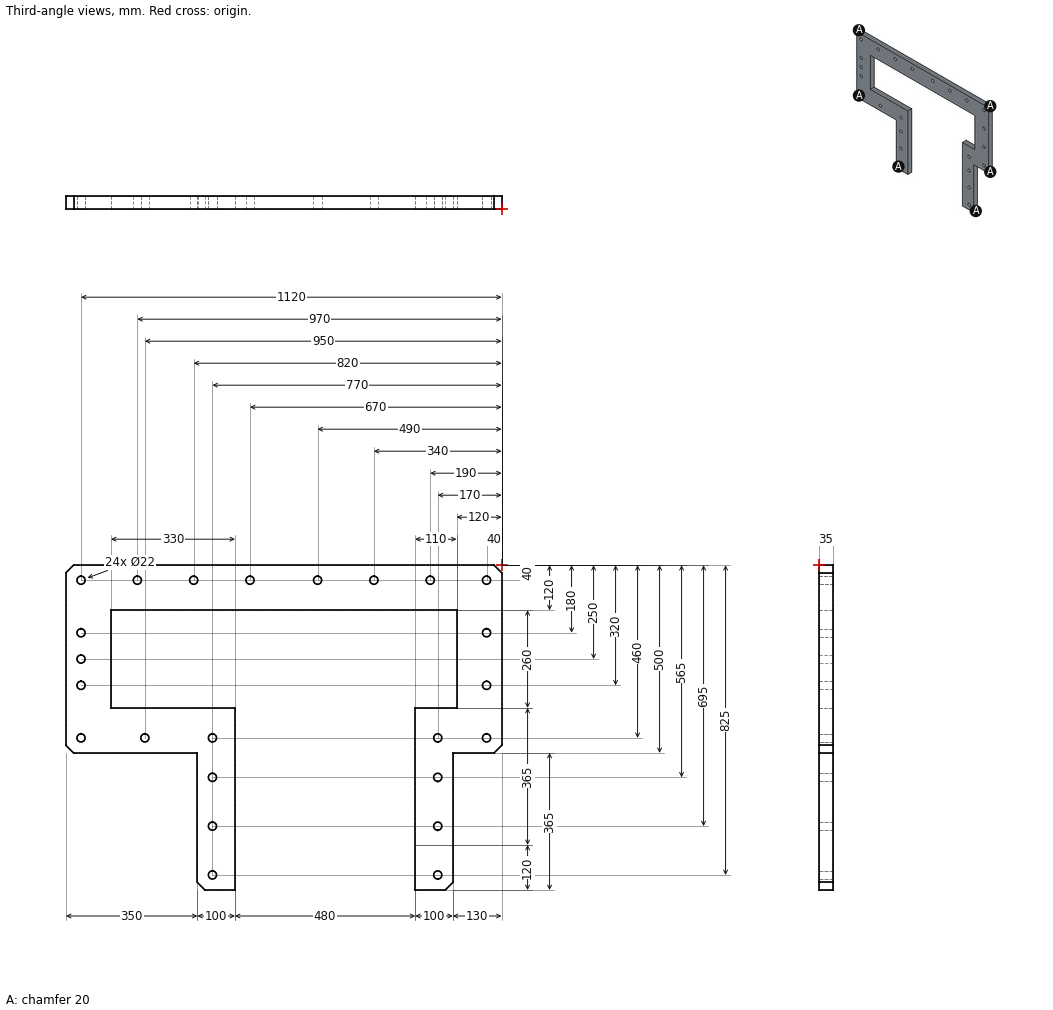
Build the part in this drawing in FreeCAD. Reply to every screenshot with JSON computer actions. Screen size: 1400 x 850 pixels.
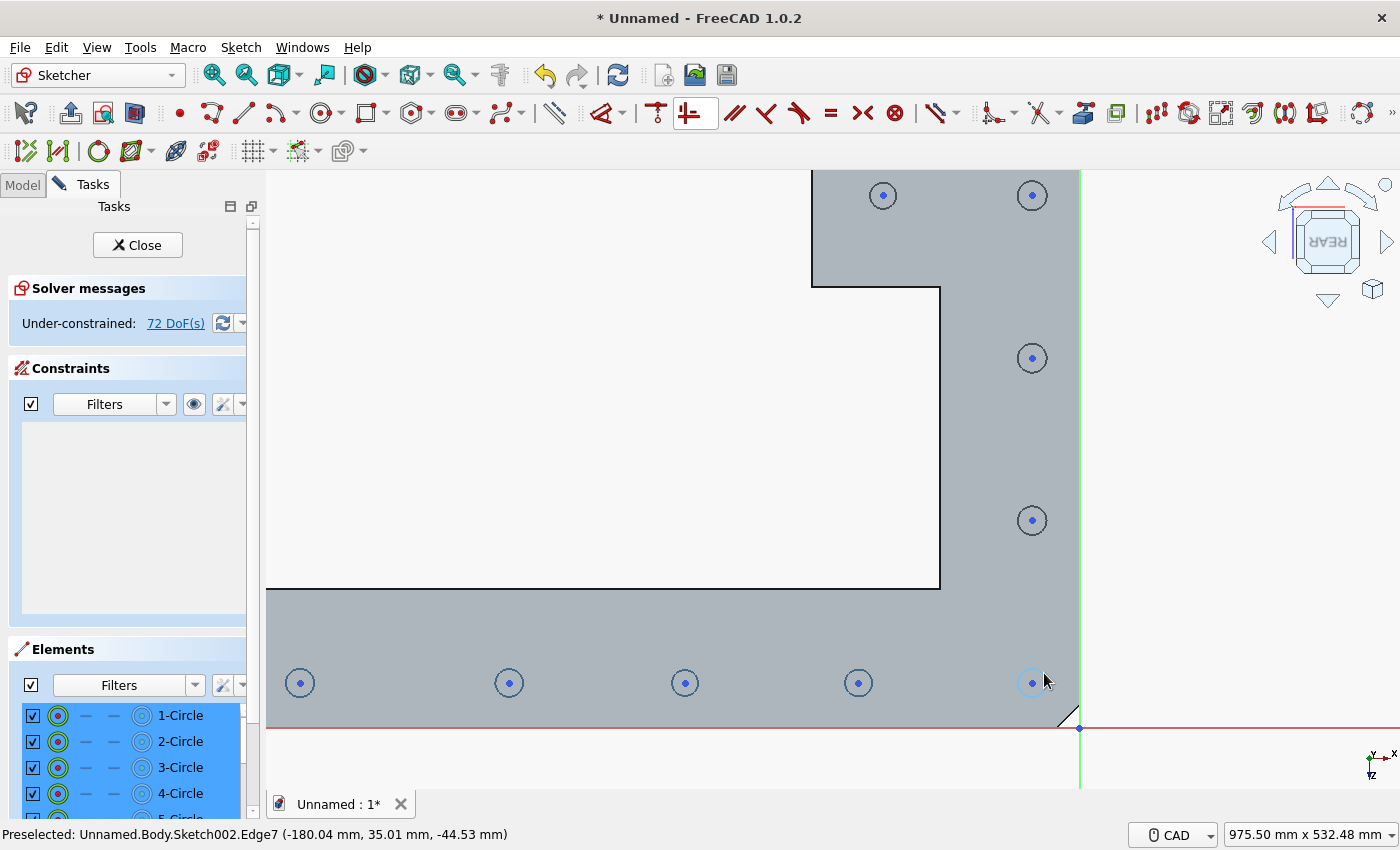
{"action": "left_click", "coordinate": [1042, 673]}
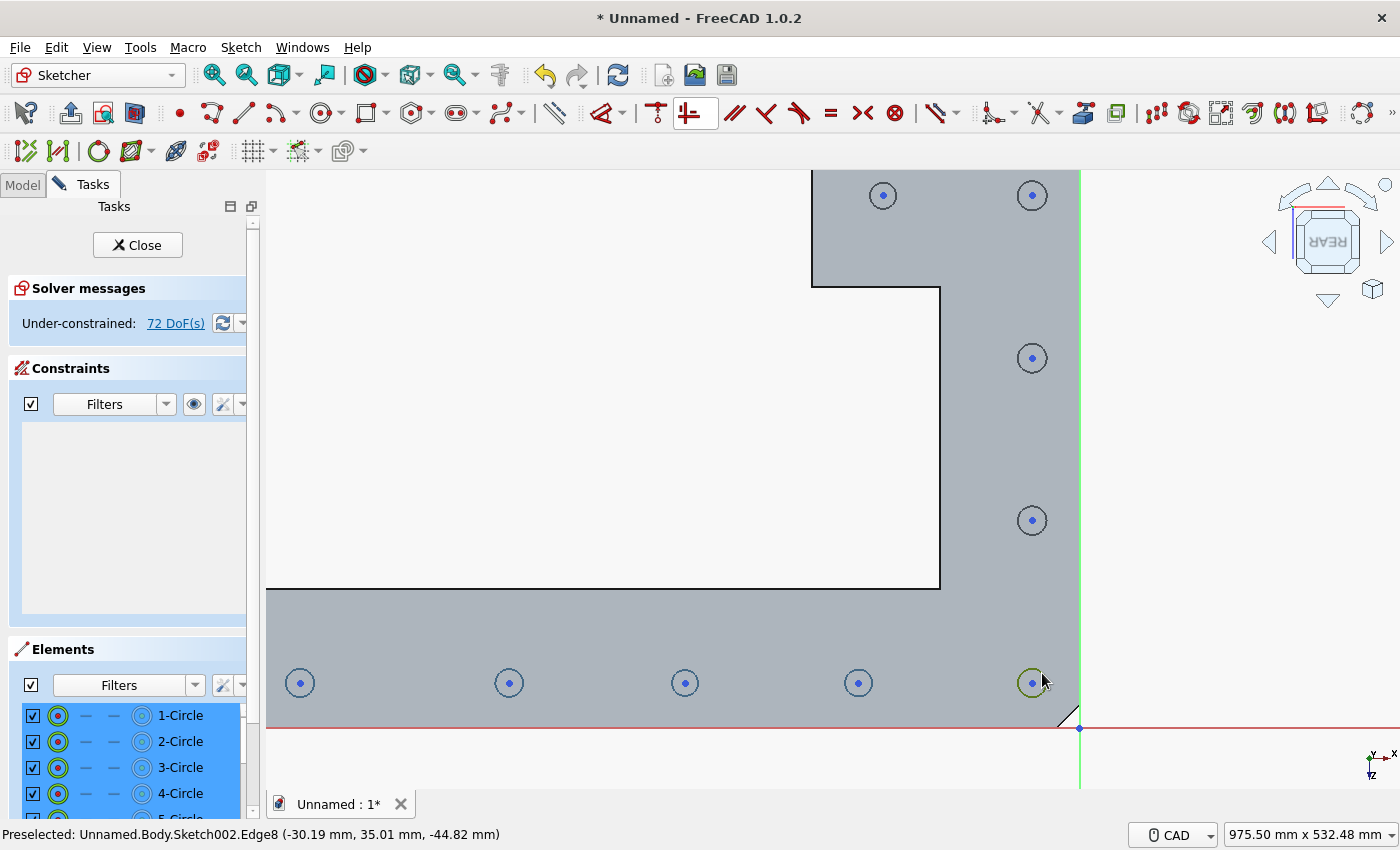
{"action": "scroll", "coordinate": [1044, 673], "scroll_direction": "down", "scroll_amount": 4}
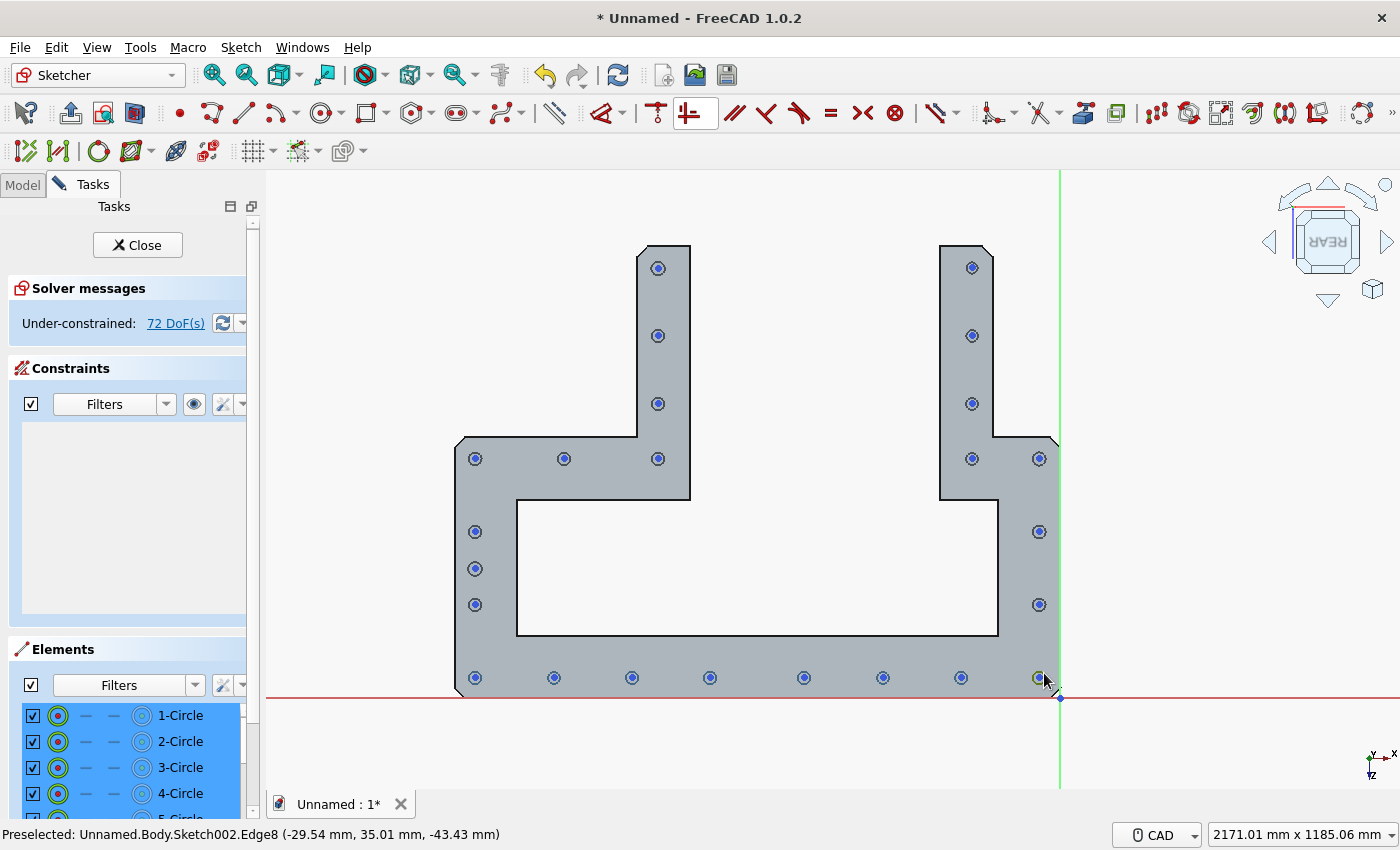
{"action": "scroll", "coordinate": [663, 264], "scroll_direction": "up", "scroll_amount": 4}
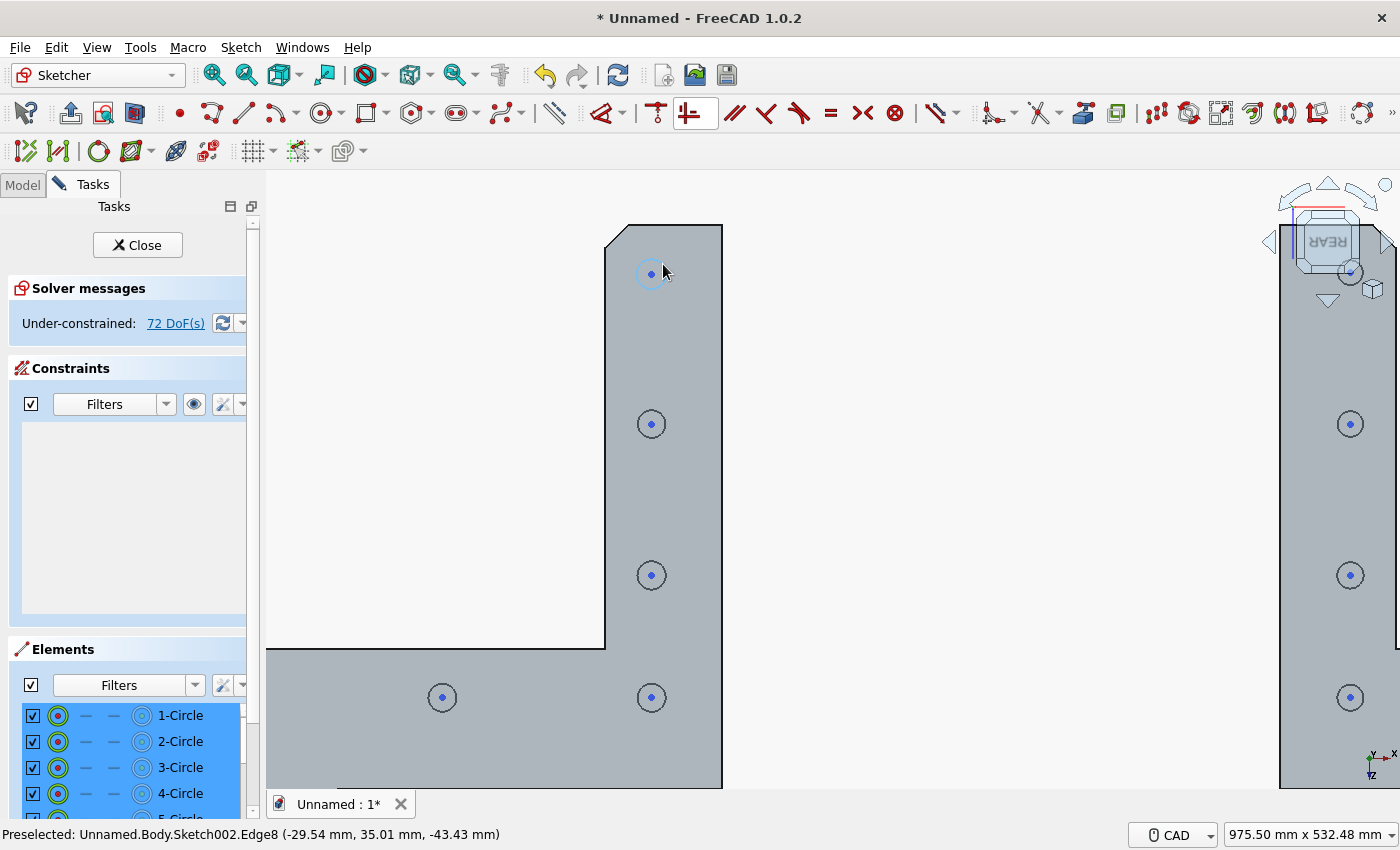
{"action": "left_click", "coordinate": [662, 264]}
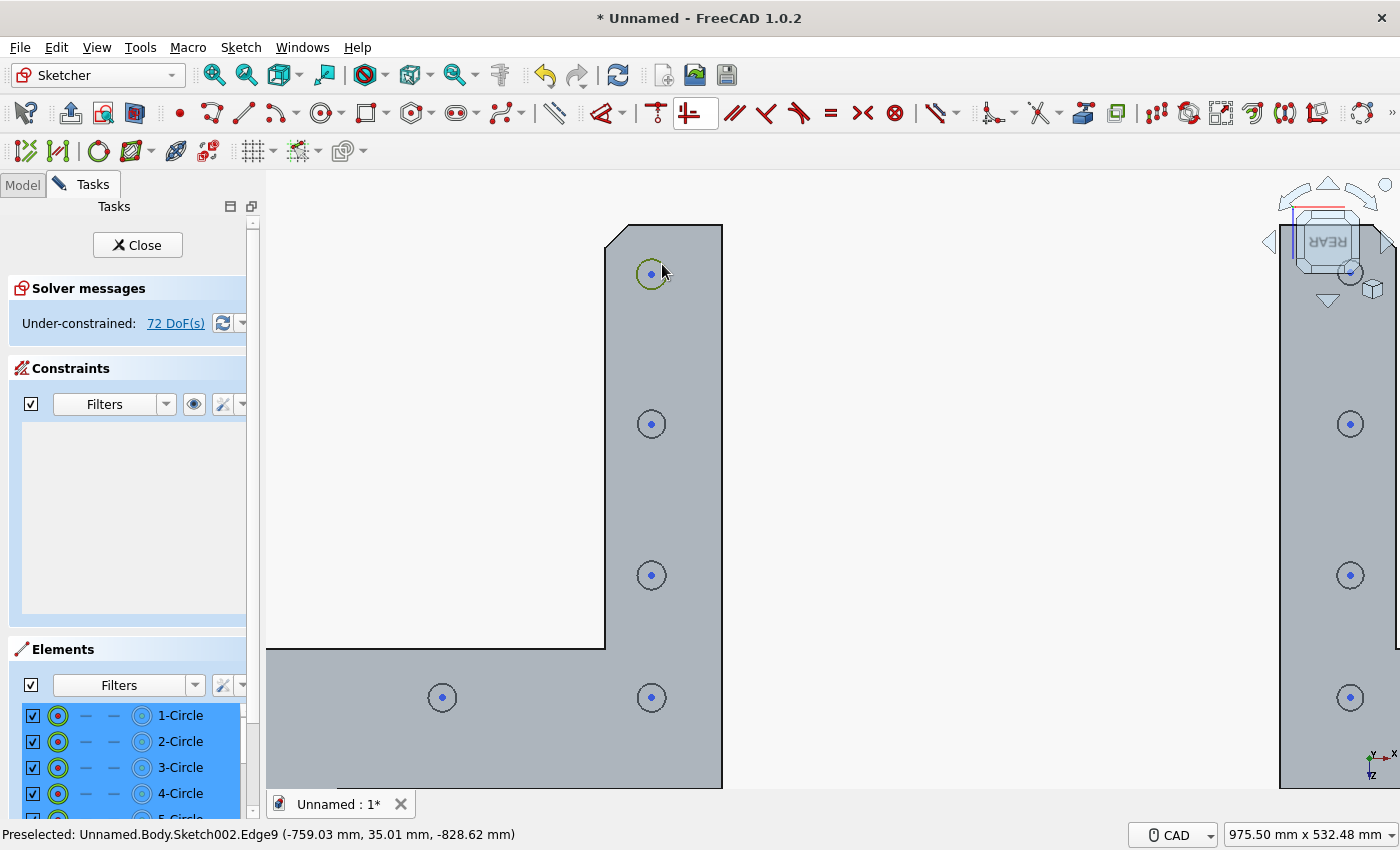
{"action": "left_click", "coordinate": [661, 414]}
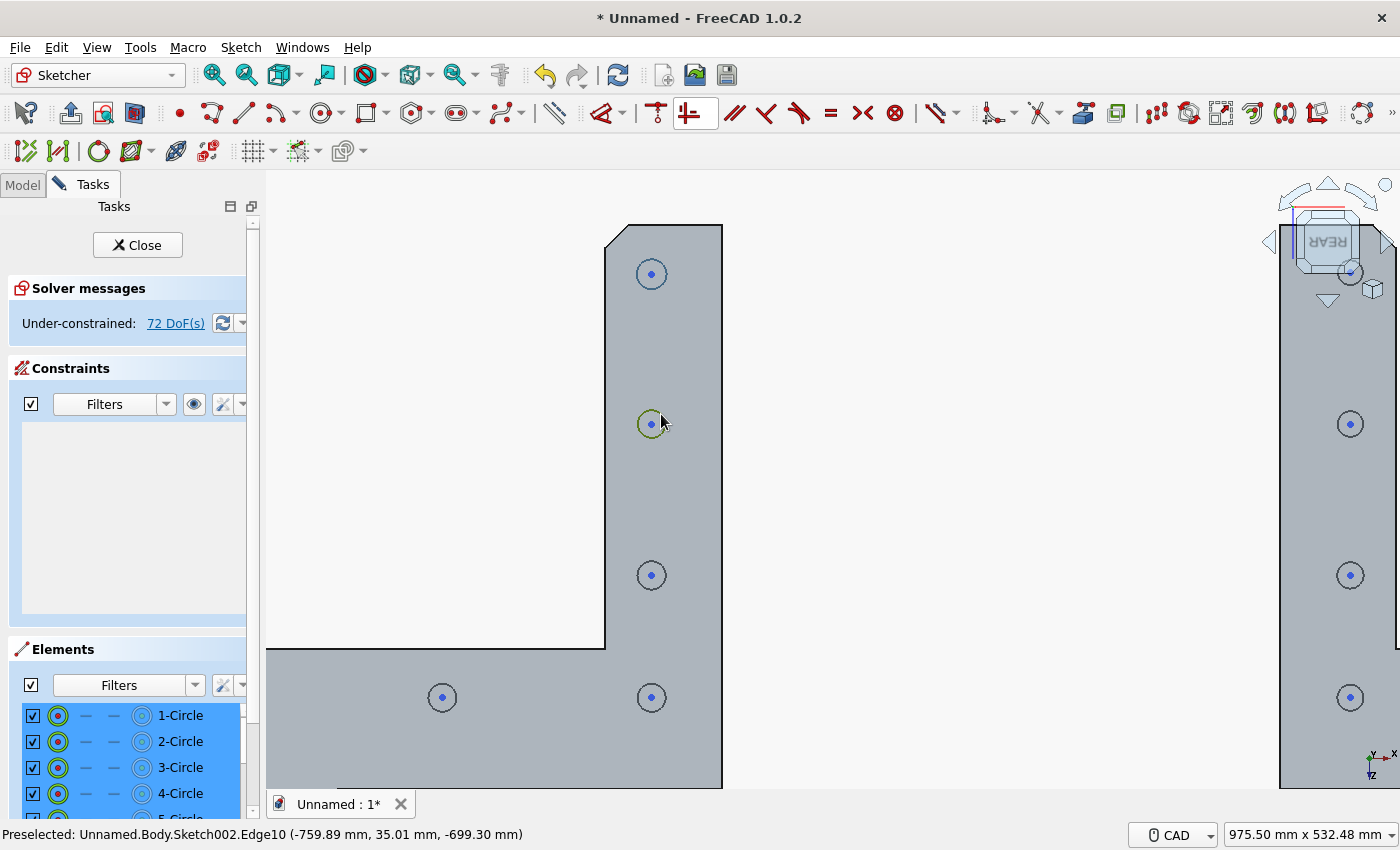
{"action": "left_click", "coordinate": [662, 565]}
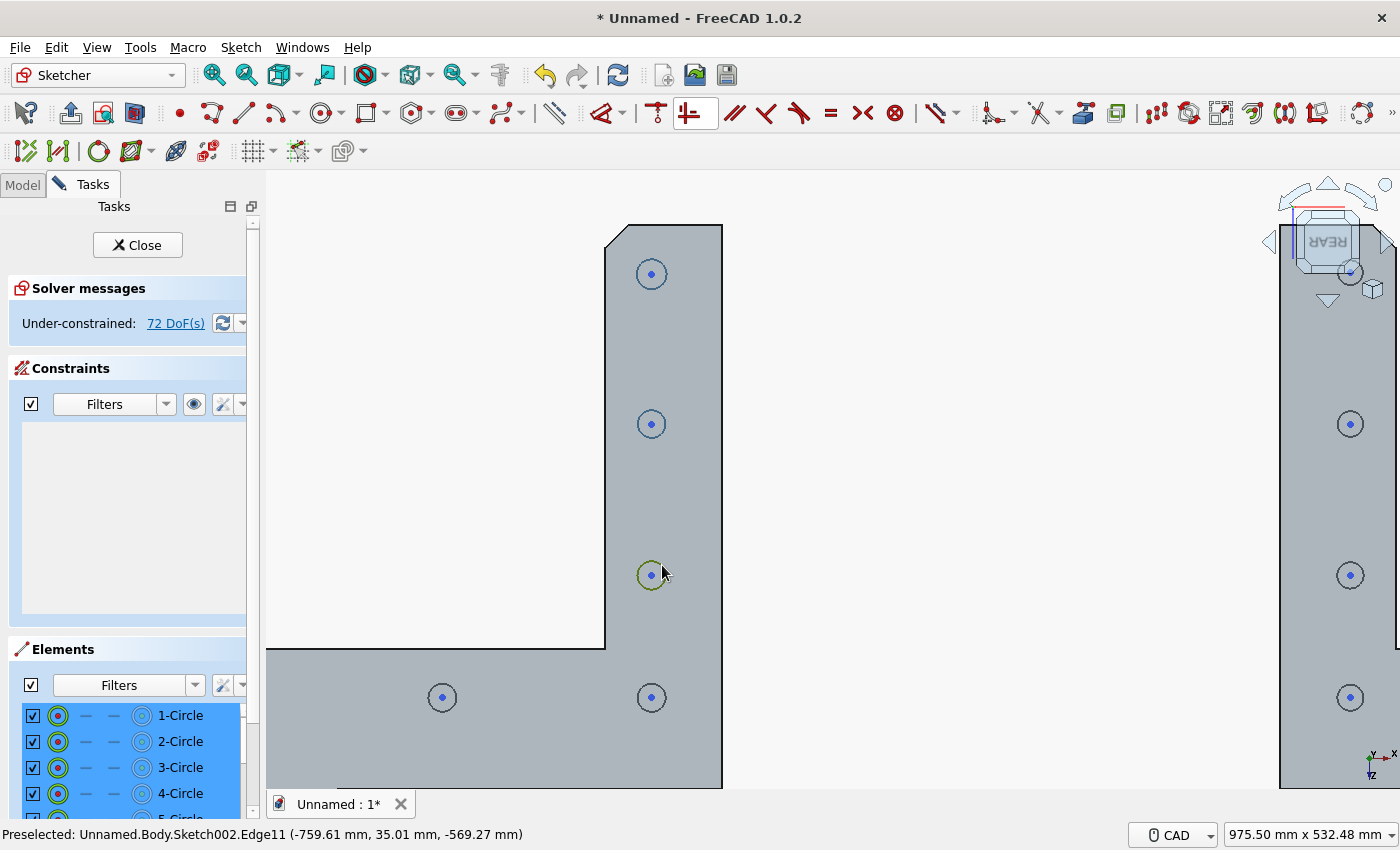
{"action": "left_click", "coordinate": [662, 688]}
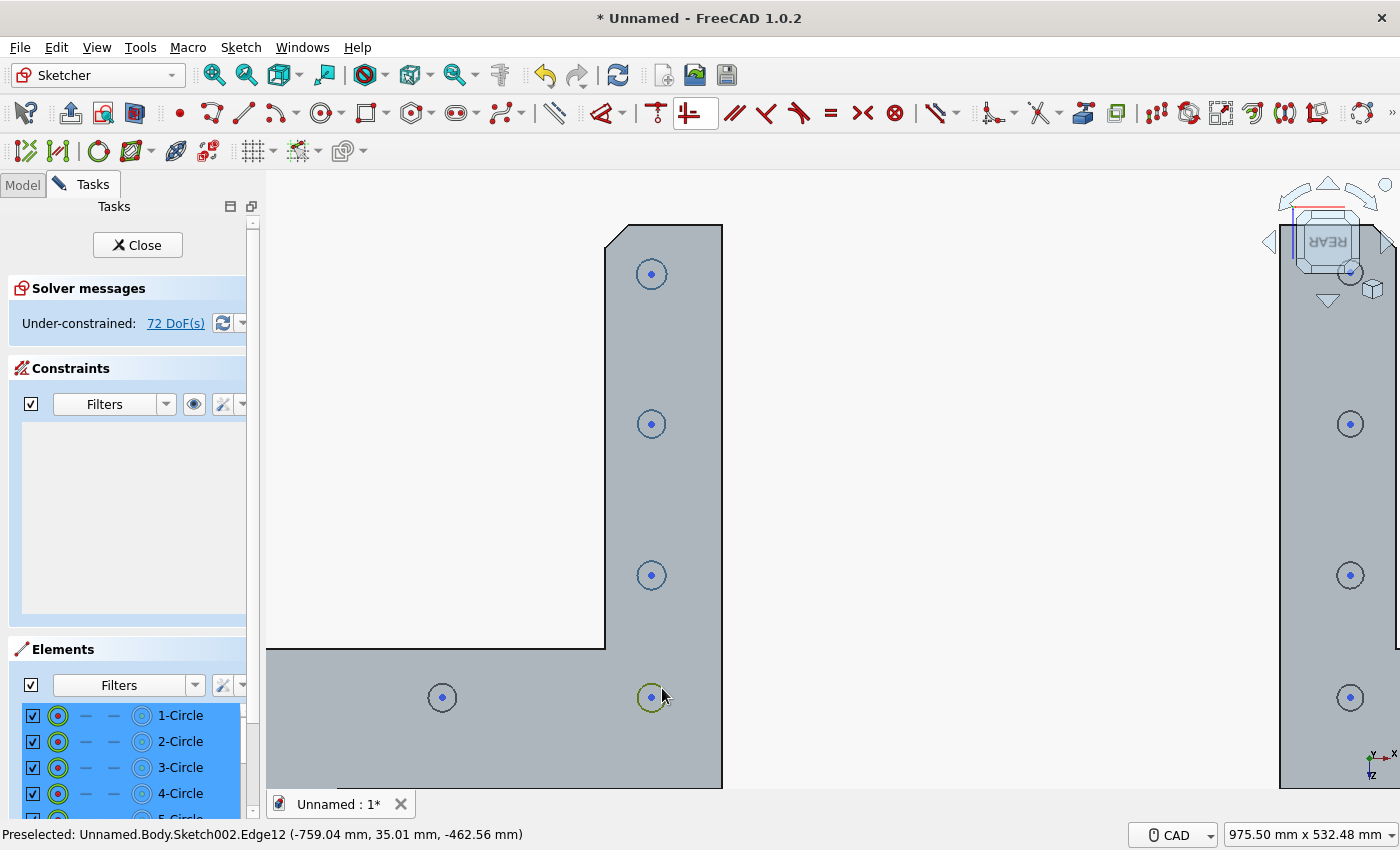
{"action": "scroll", "coordinate": [662, 263], "scroll_direction": "down", "scroll_amount": 4}